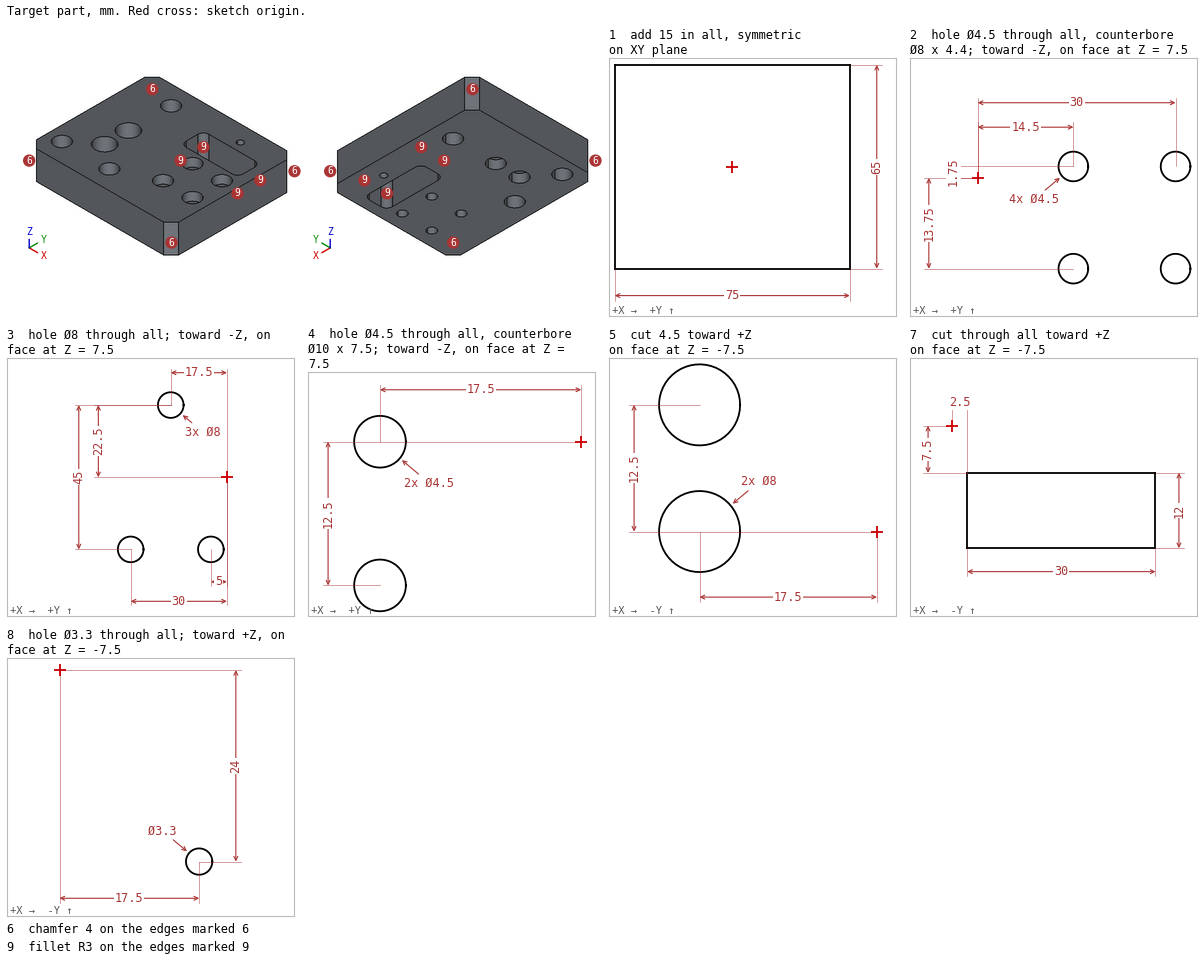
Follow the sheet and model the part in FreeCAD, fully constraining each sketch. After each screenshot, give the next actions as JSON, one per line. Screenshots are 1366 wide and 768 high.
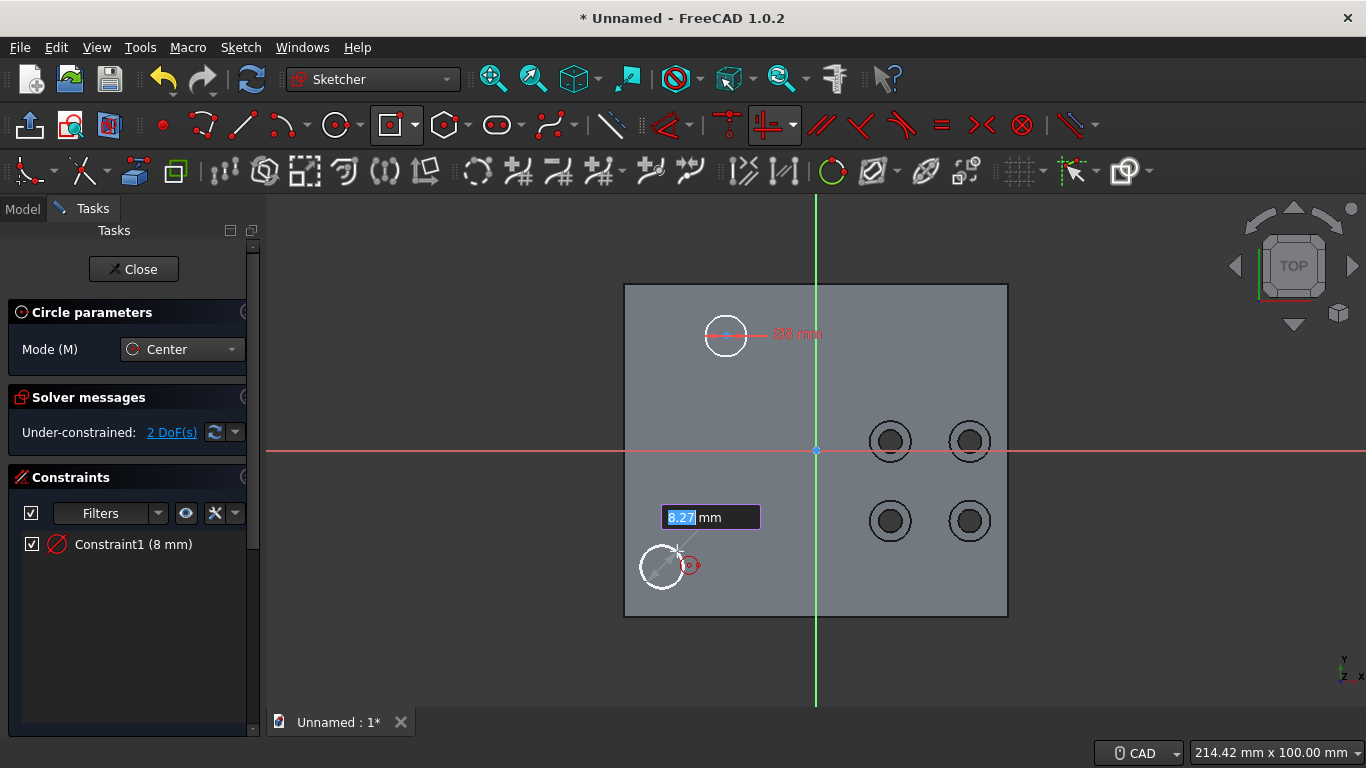
{"action": "type", "text": "8"}
{"action": "key", "text": "Return"}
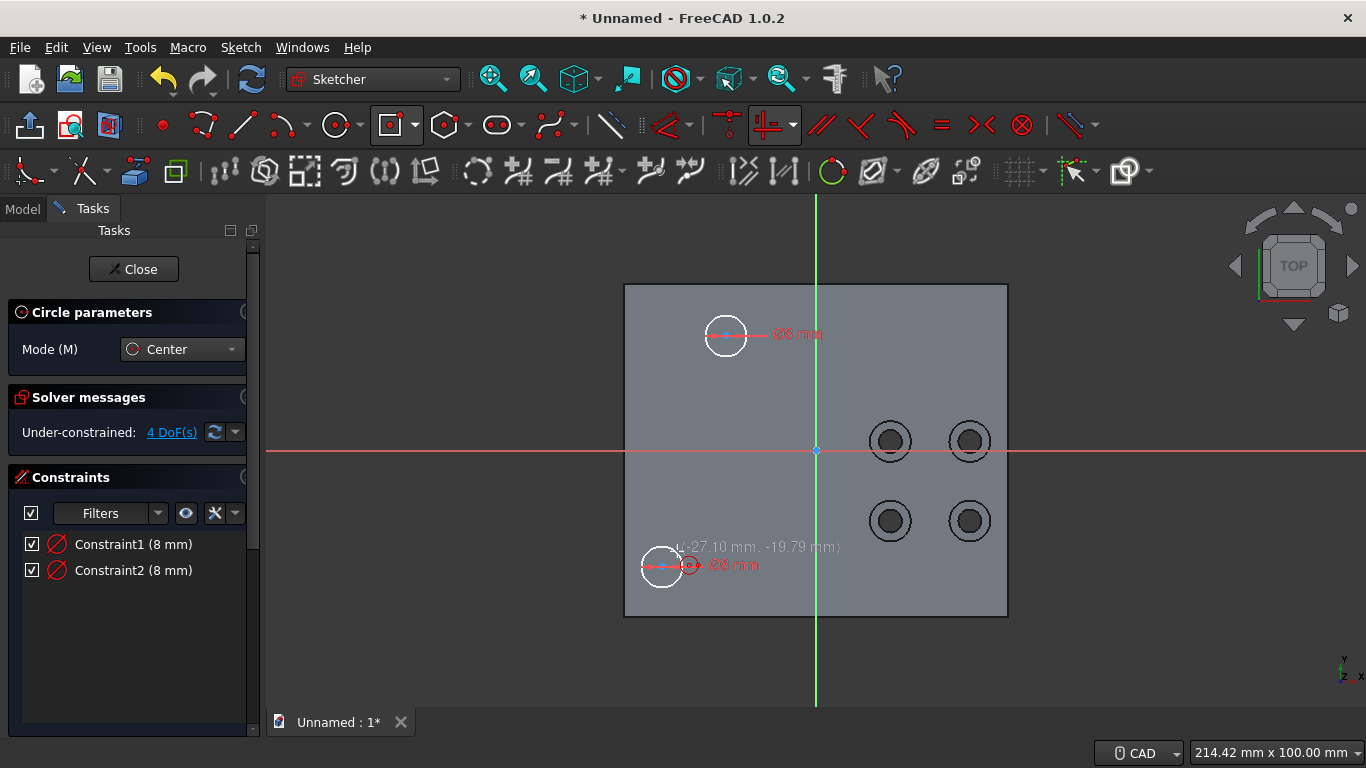
{"action": "left_click", "coordinate": [790, 566]}
{"action": "mouse_move", "coordinate": [776, 551]}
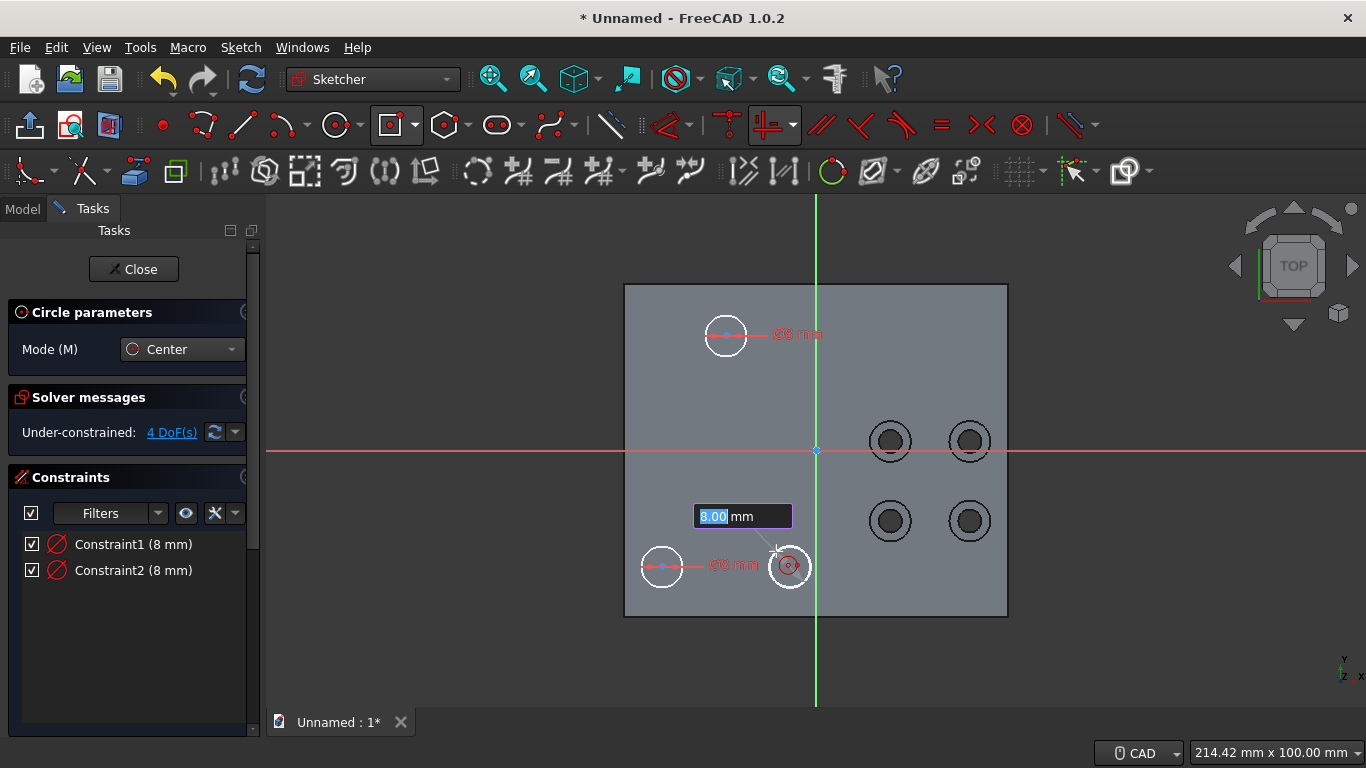
{"action": "type", "text": "8"}
{"action": "key", "text": "Return"}
{"action": "key", "text": "Escape"}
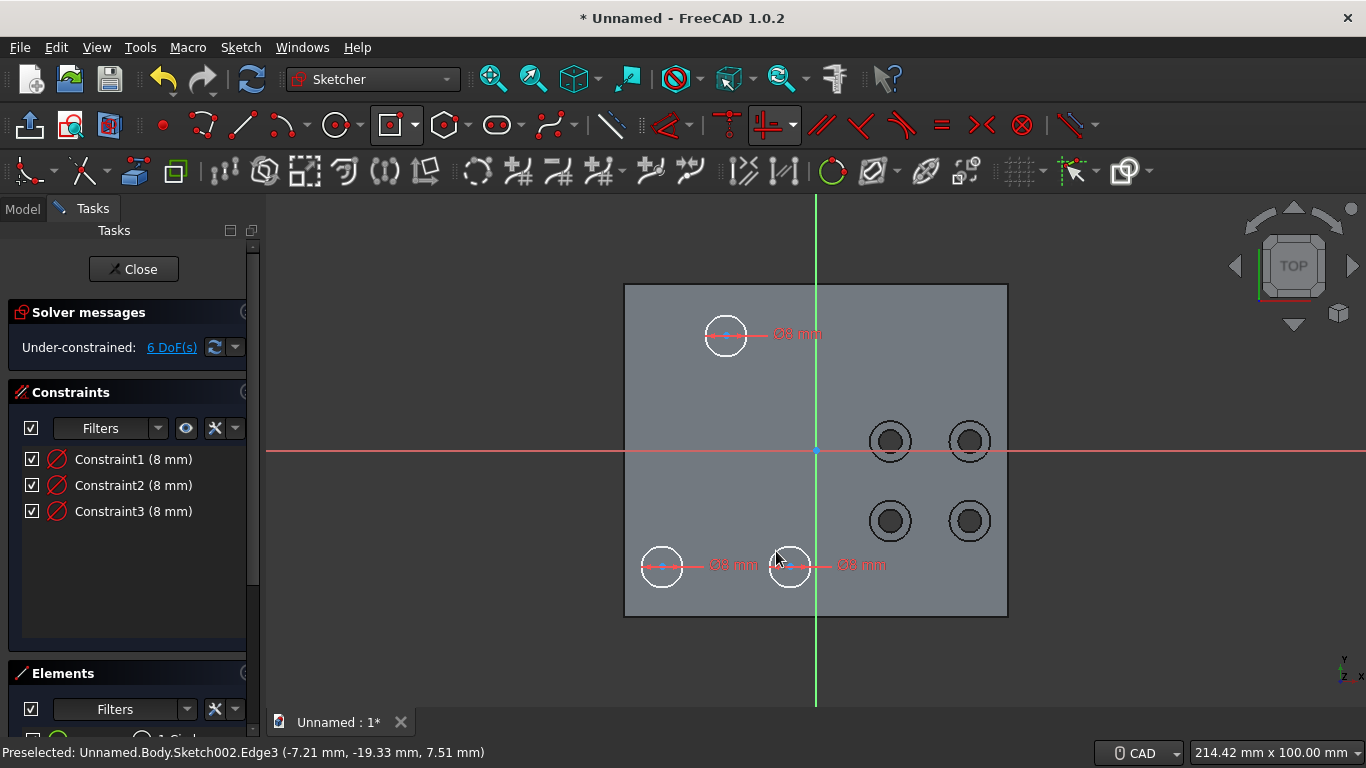
{"action": "left_click", "coordinate": [662, 567]}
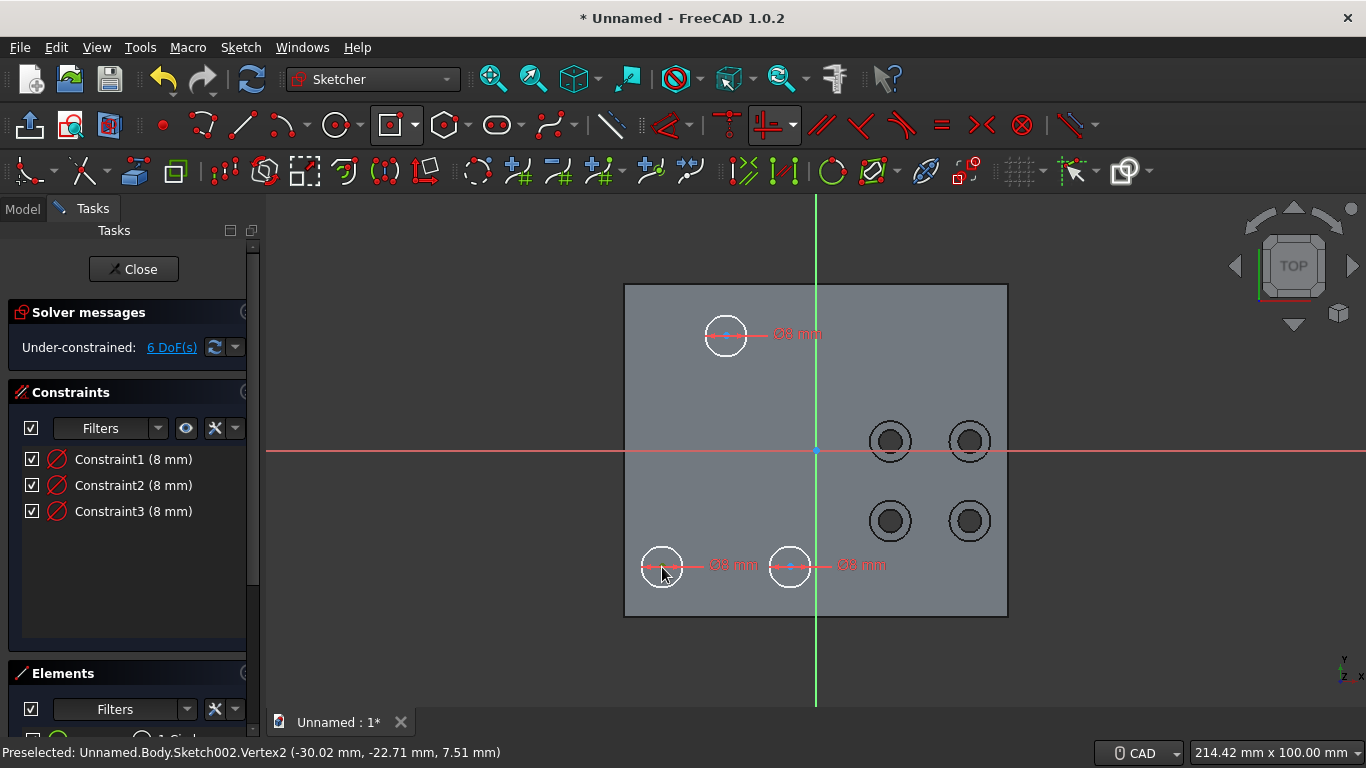
{"action": "left_click", "coordinate": [790, 567]}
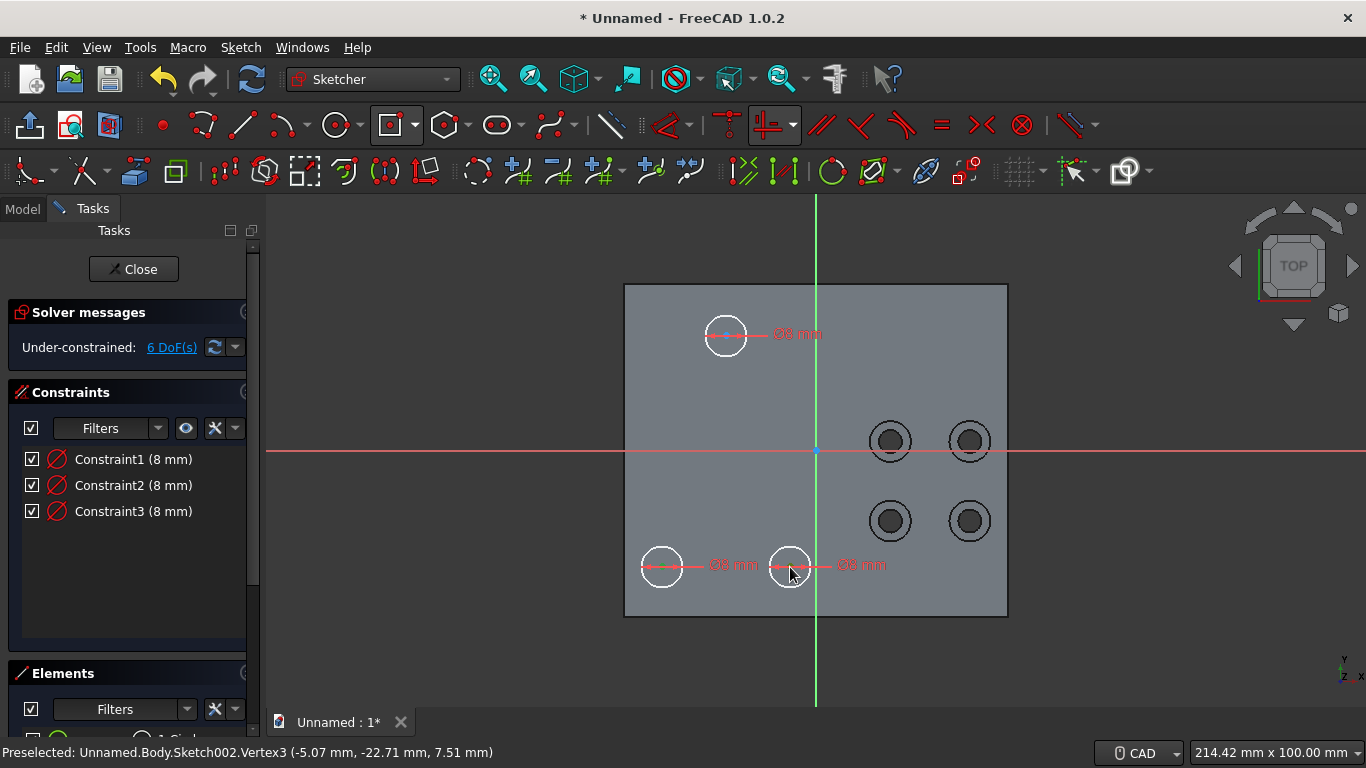
{"action": "key", "text": "h"}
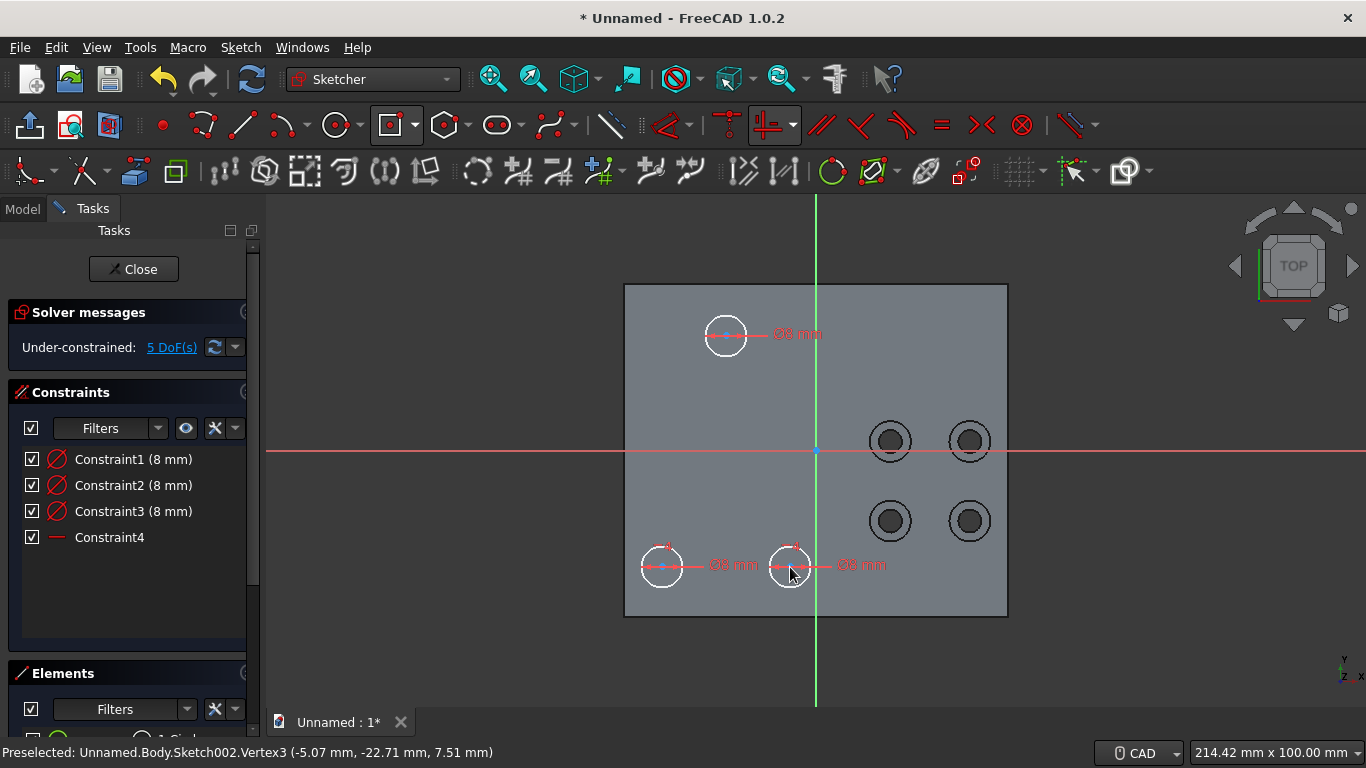
{"action": "scroll", "coordinate": [790, 567], "scroll_direction": "up", "scroll_amount": 3}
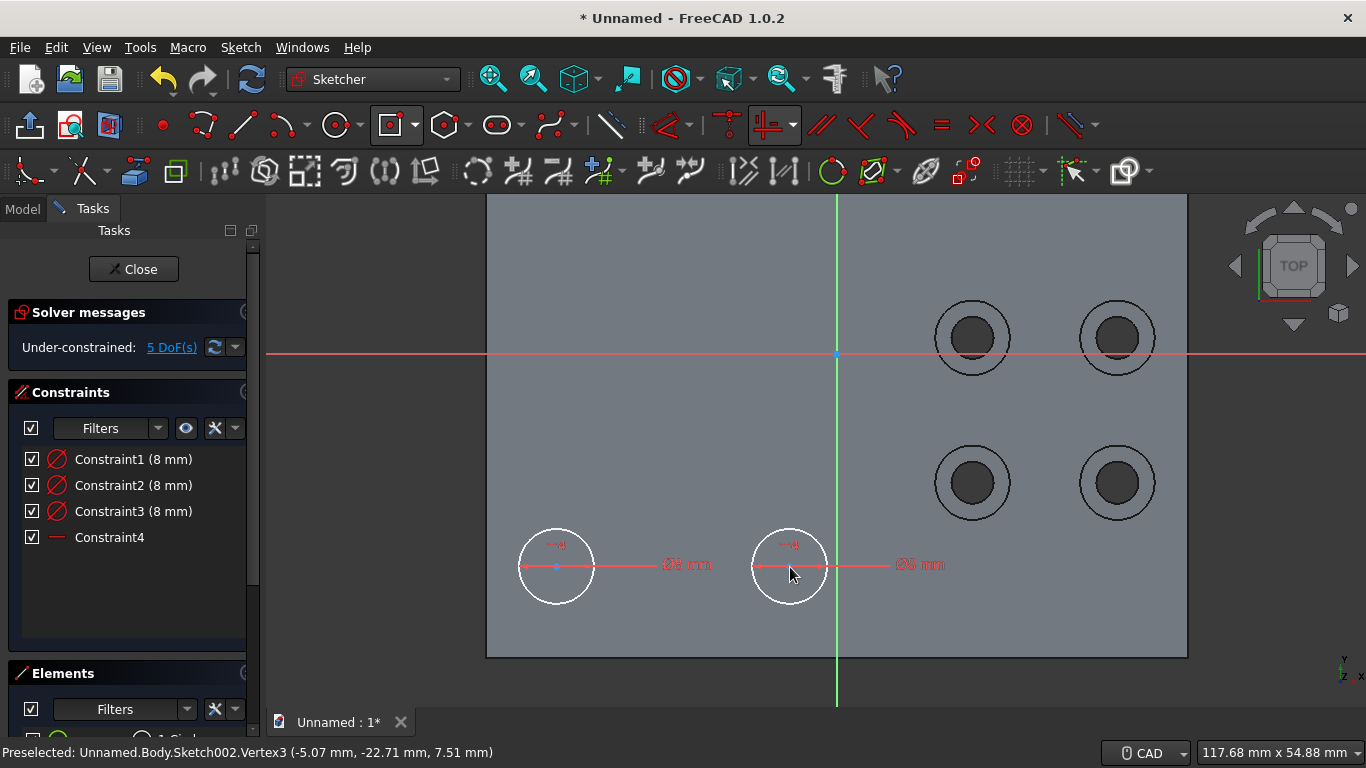
{"action": "left_click", "coordinate": [790, 566]}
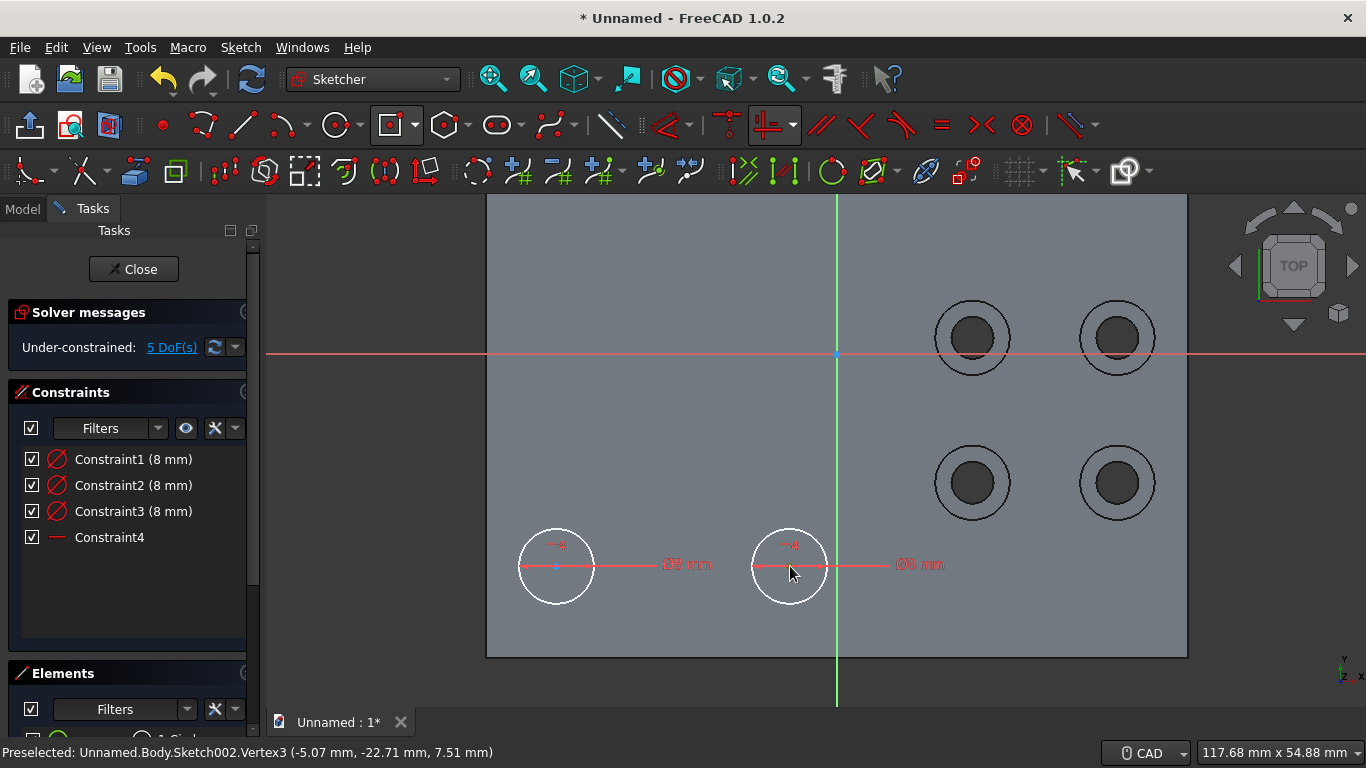
{"action": "key", "text": "l"}